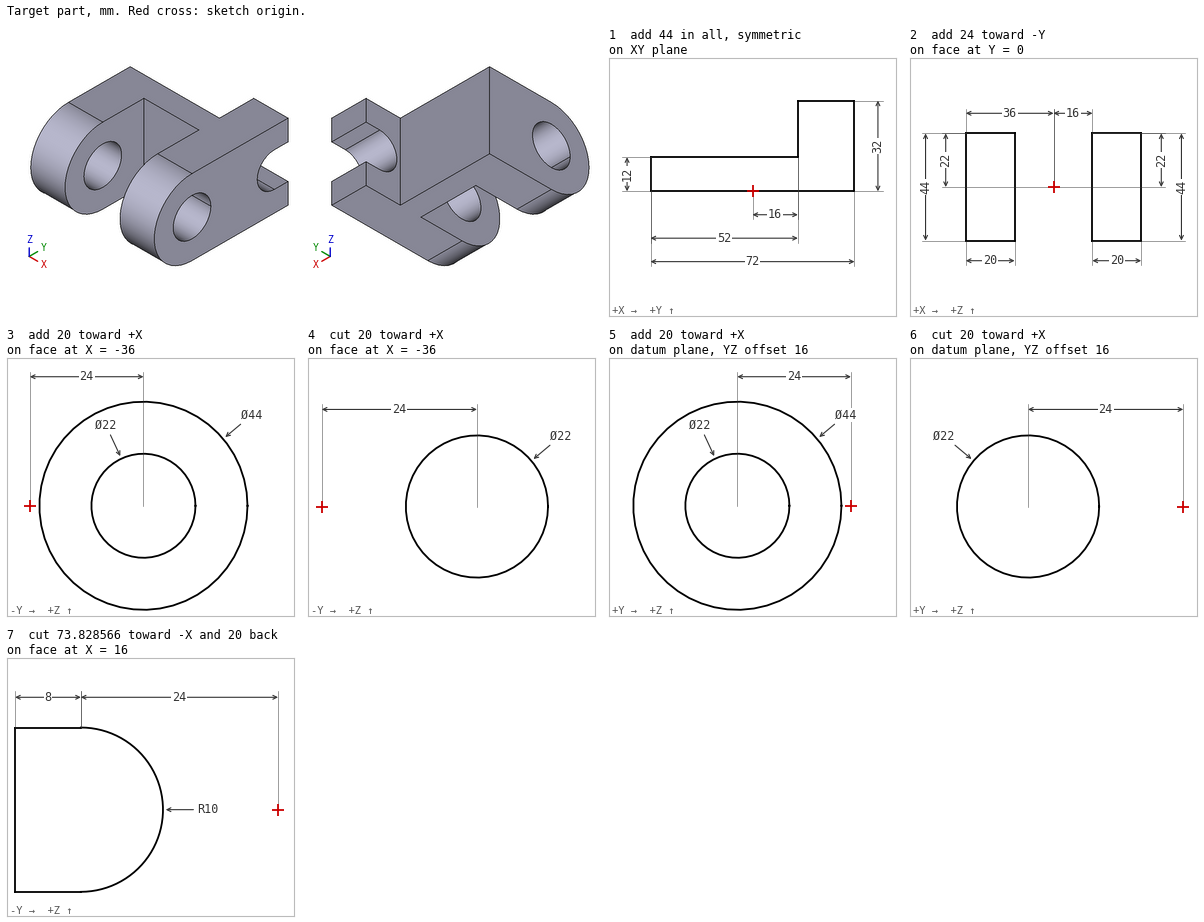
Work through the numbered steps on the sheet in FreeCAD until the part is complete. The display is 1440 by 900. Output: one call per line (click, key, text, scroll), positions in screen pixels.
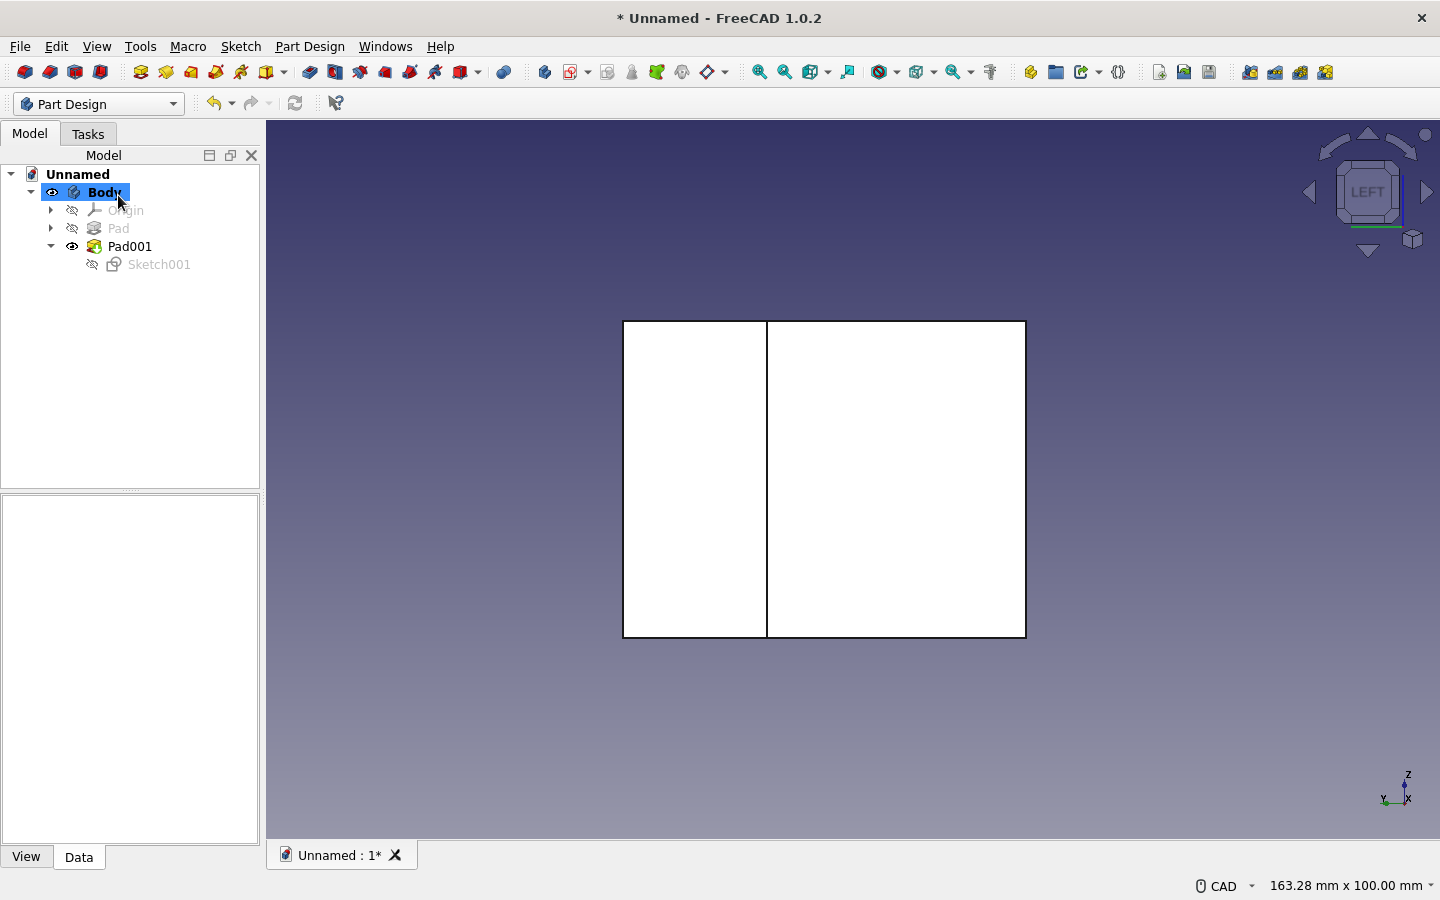
click(760, 72)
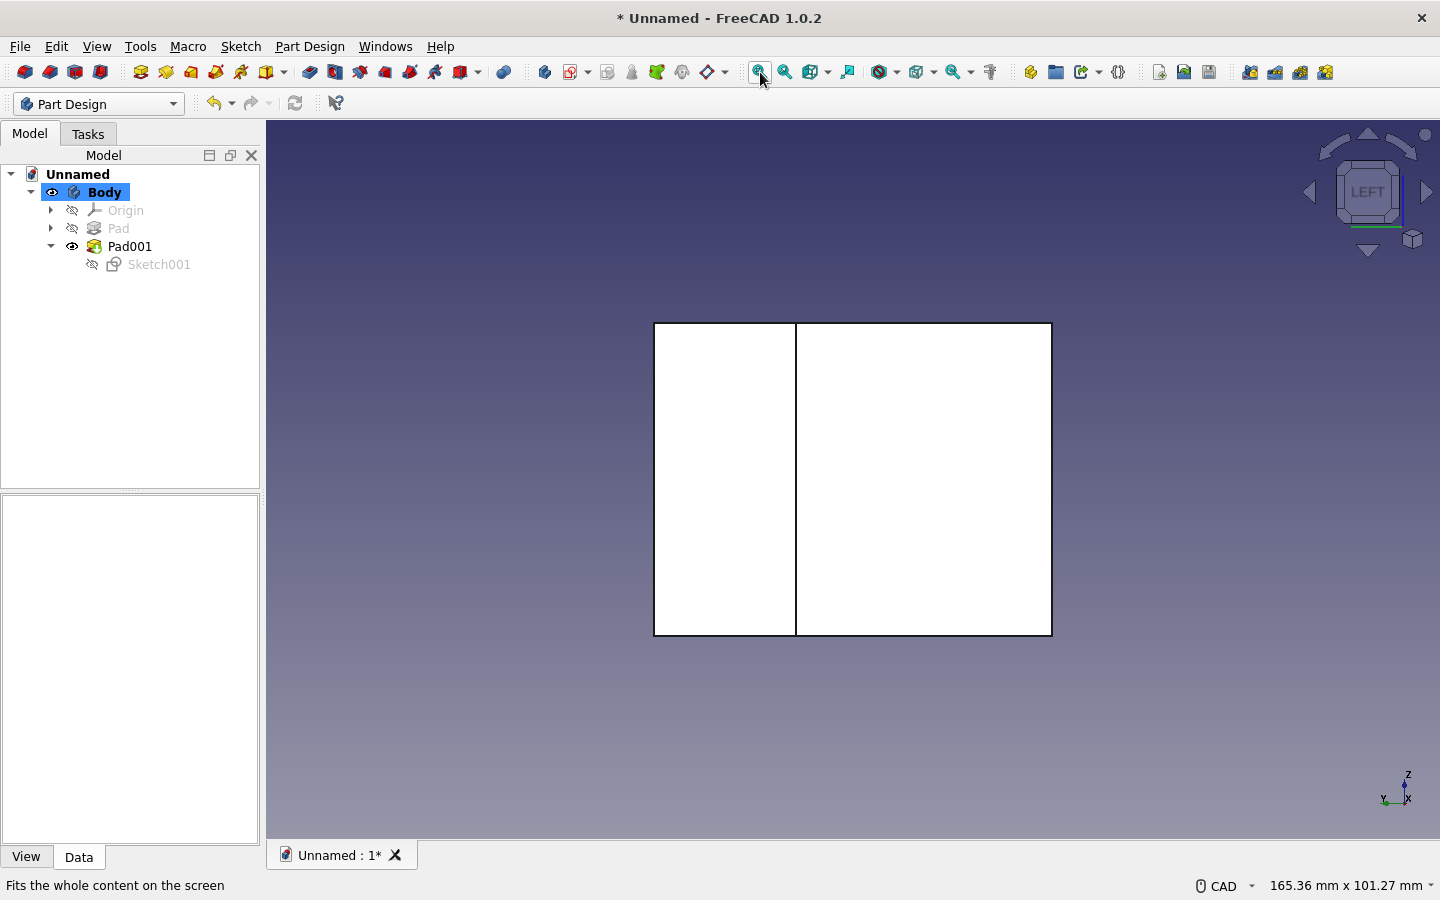
click(924, 478)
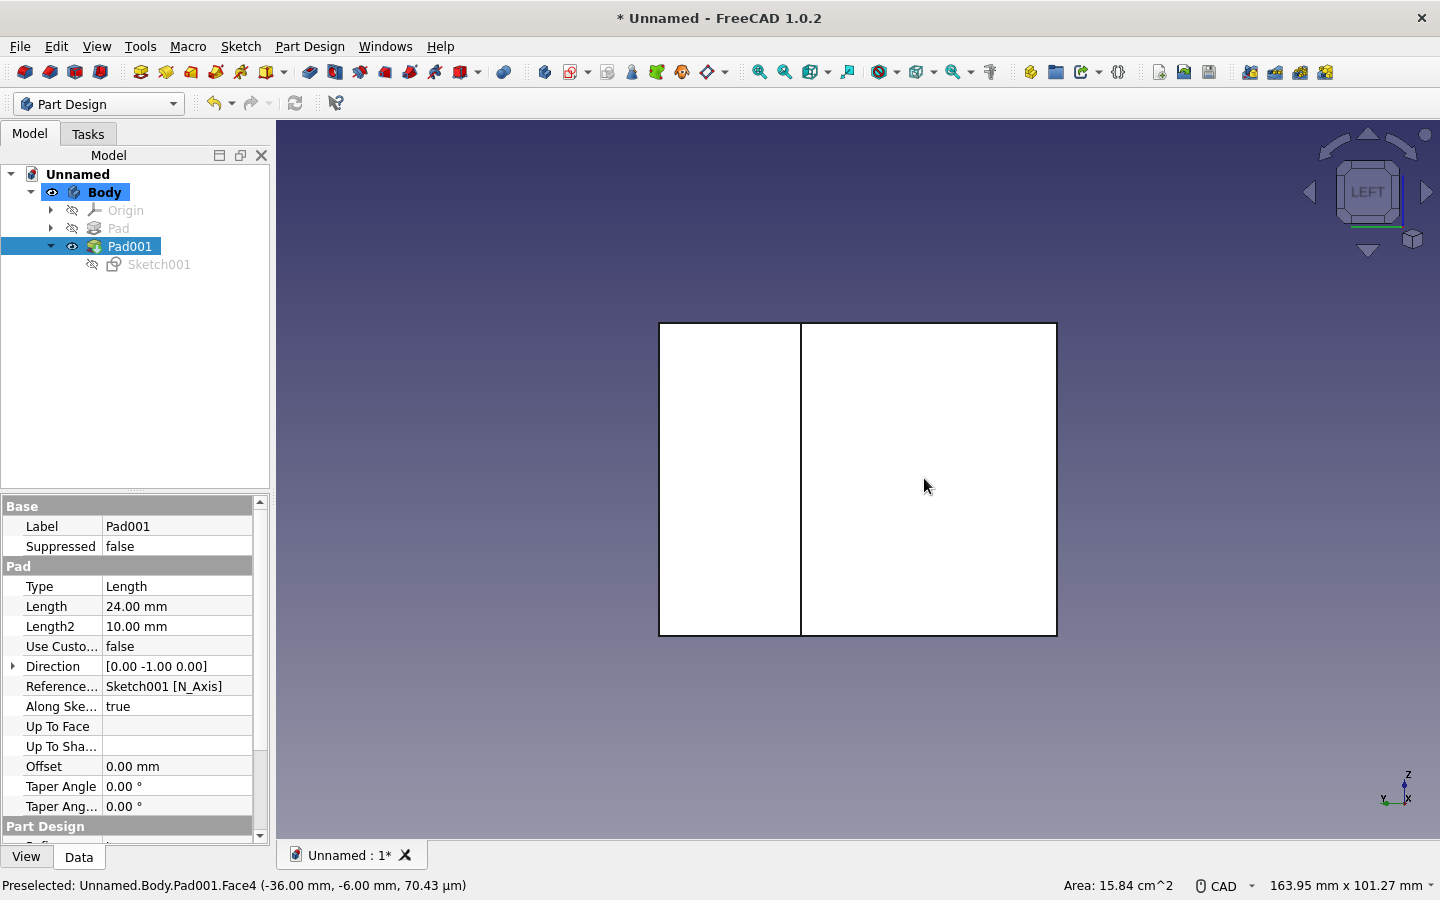
click(570, 72)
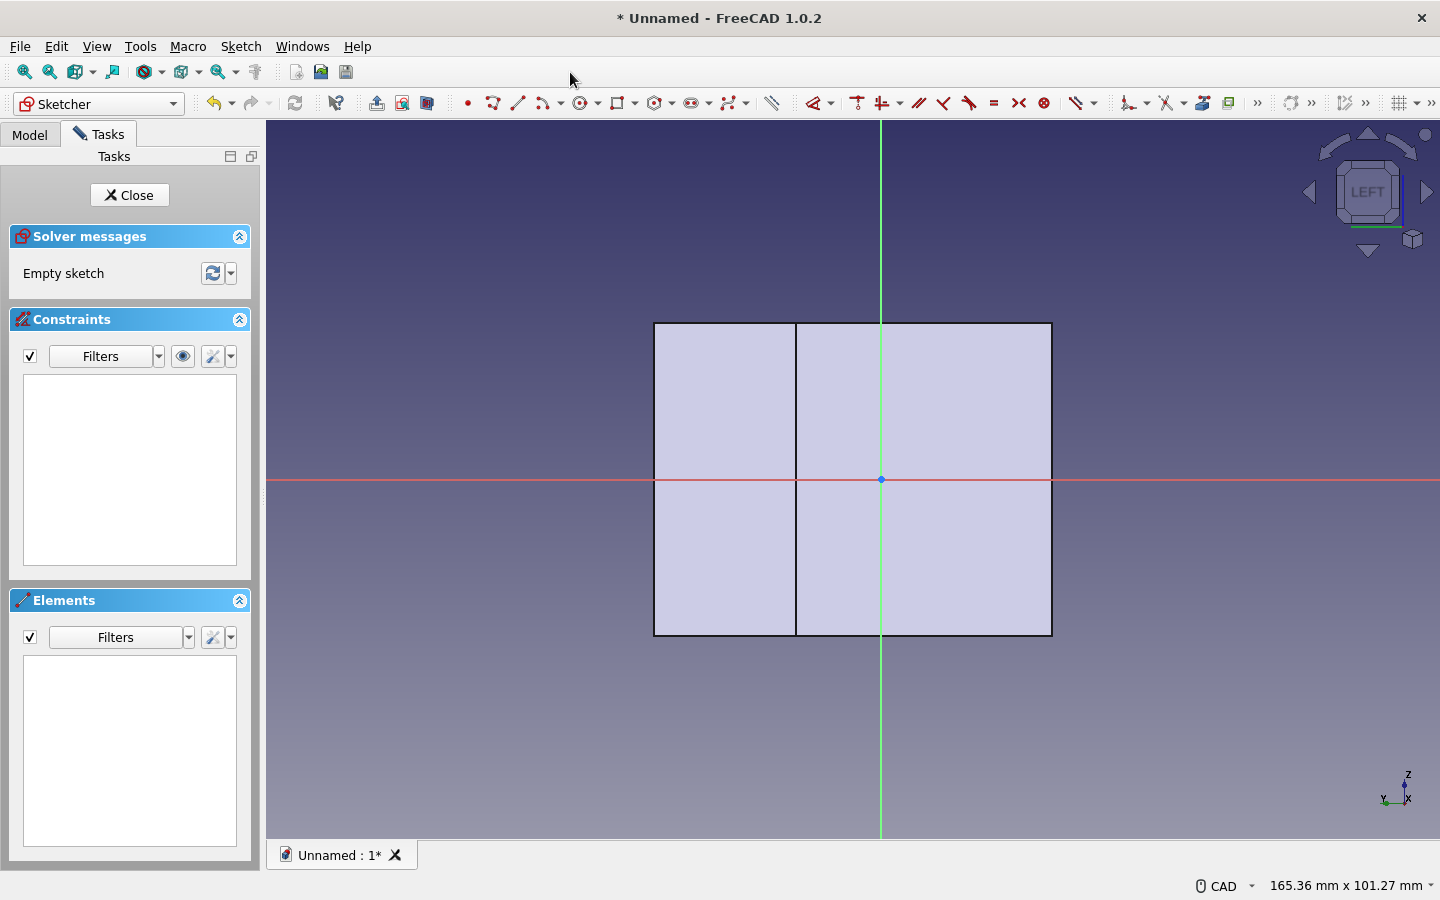
scroll(1275, 480, up, 2)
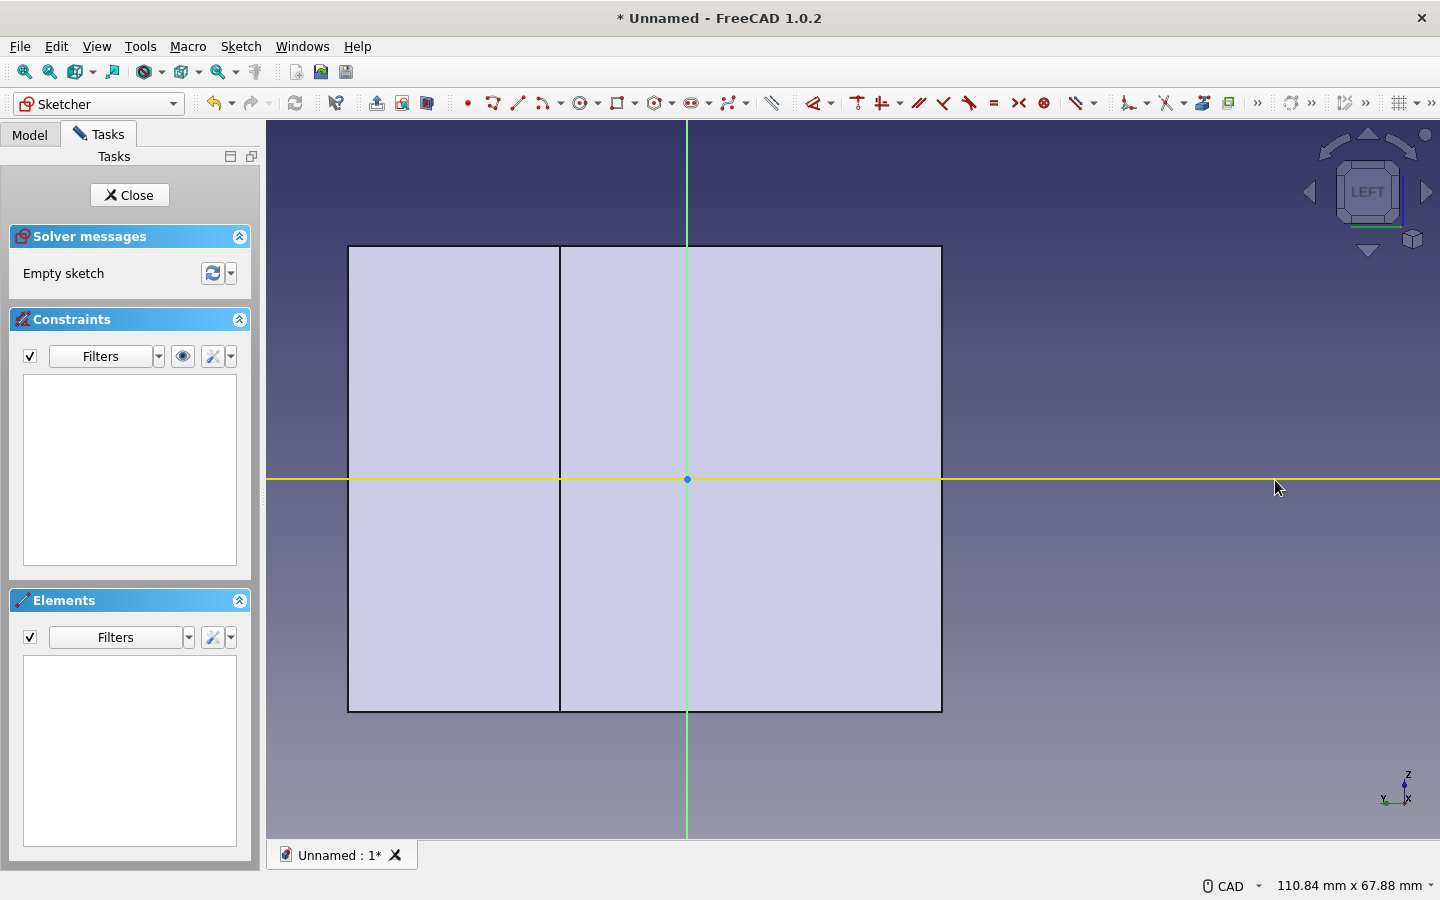
click(580, 104)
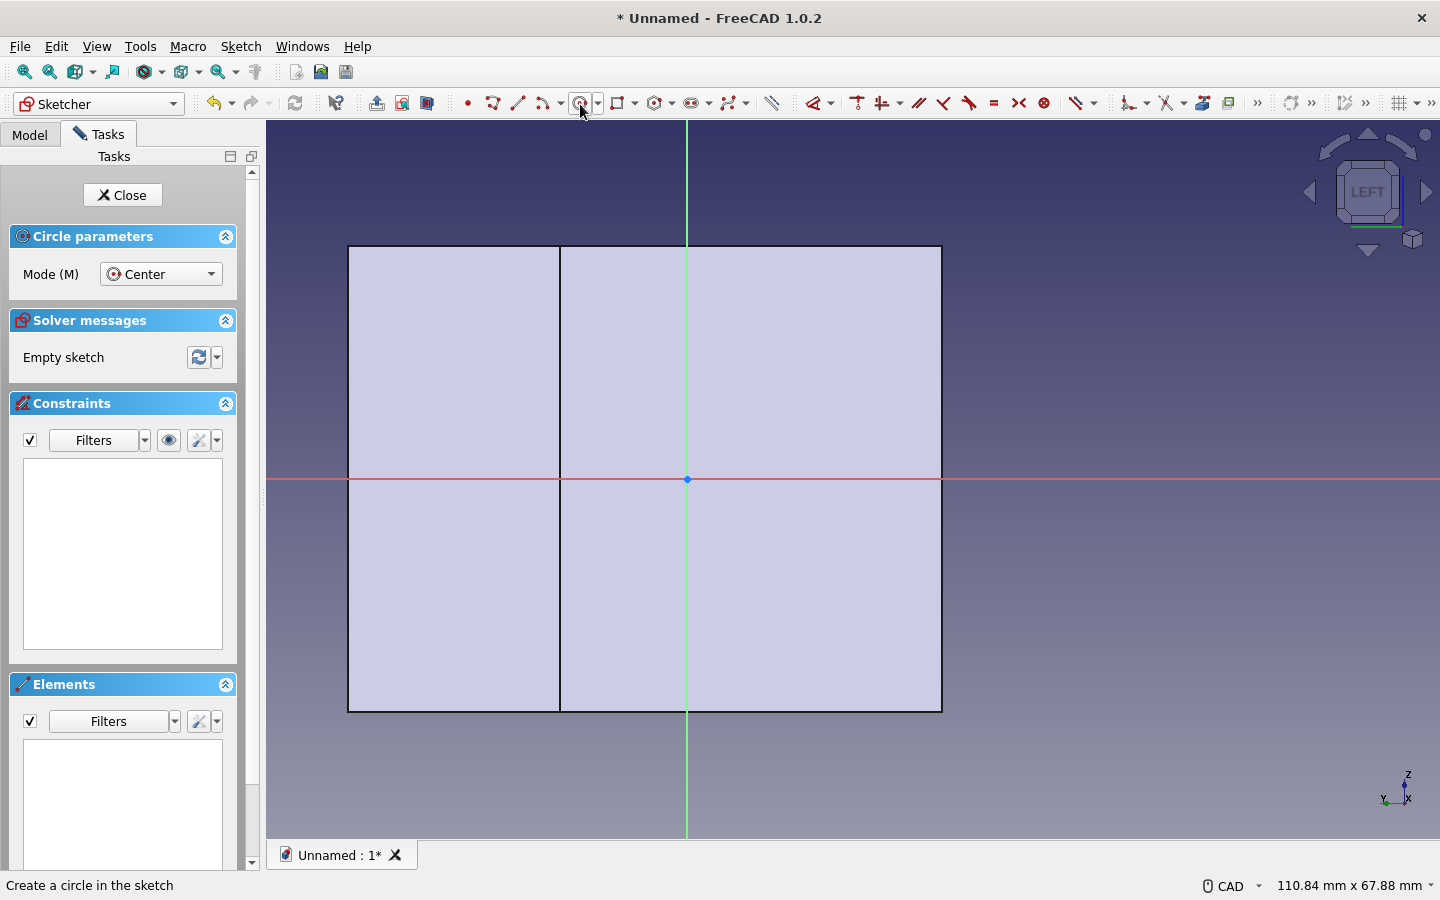
click(942, 479)
click(1106, 314)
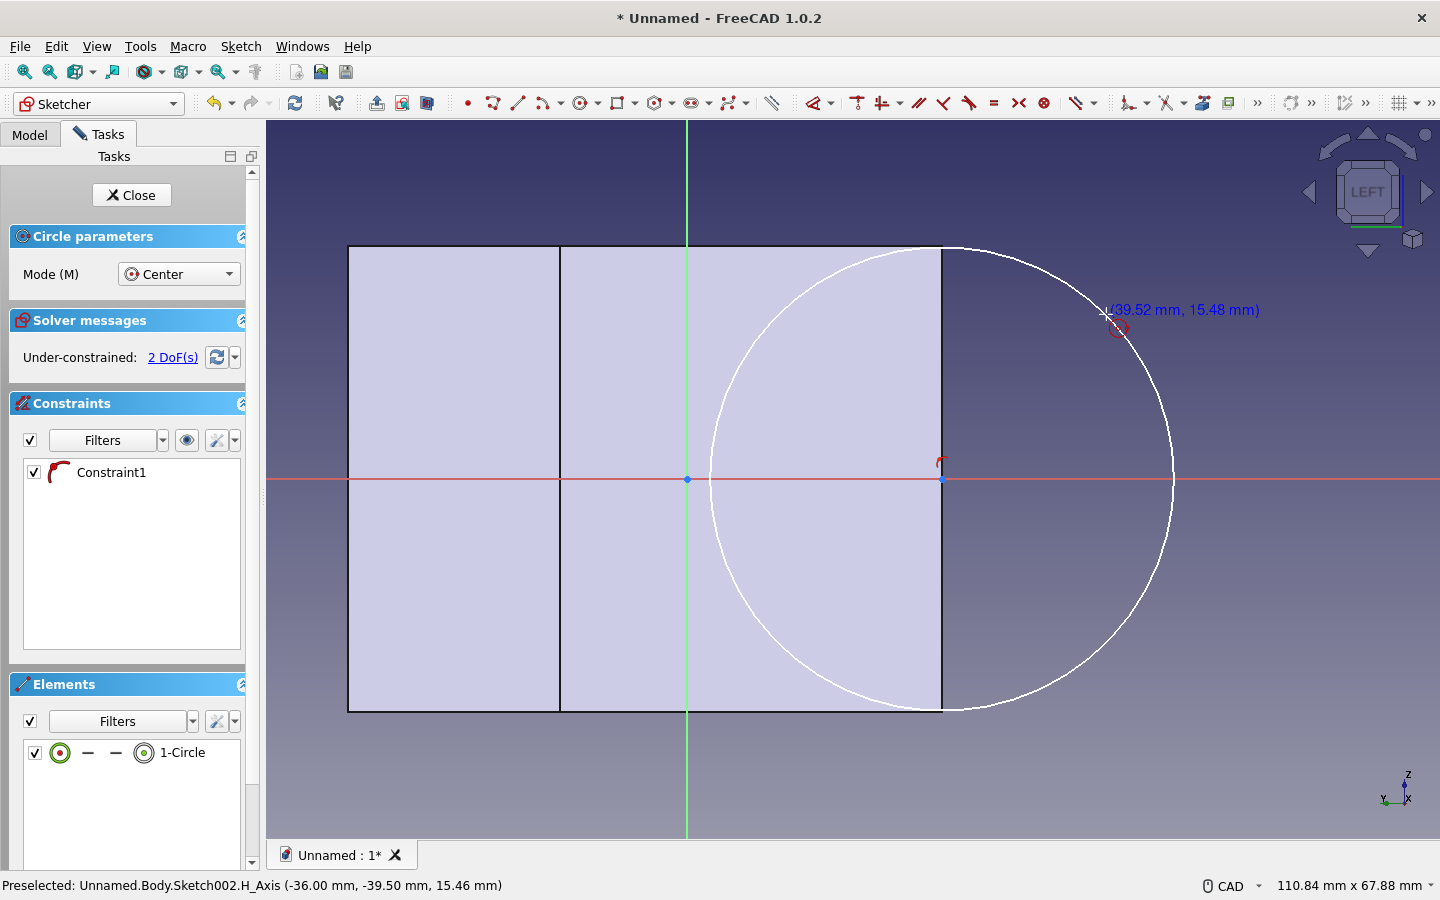
click(942, 479)
click(1024, 397)
key(Escape)